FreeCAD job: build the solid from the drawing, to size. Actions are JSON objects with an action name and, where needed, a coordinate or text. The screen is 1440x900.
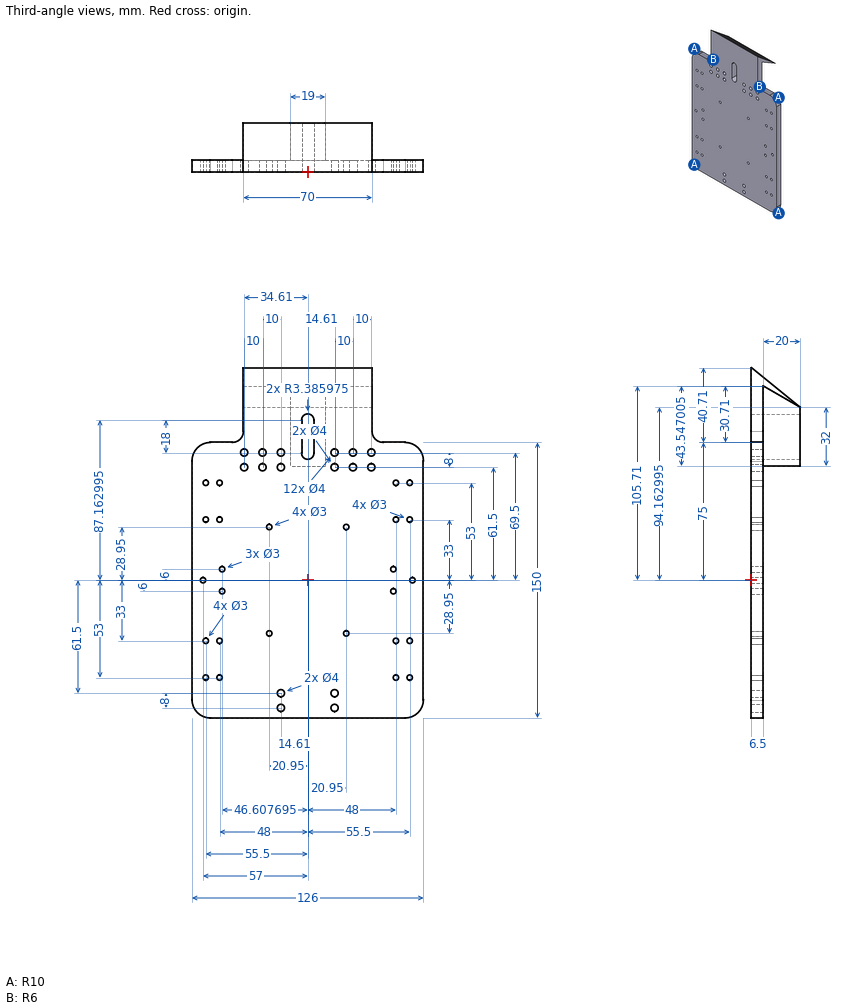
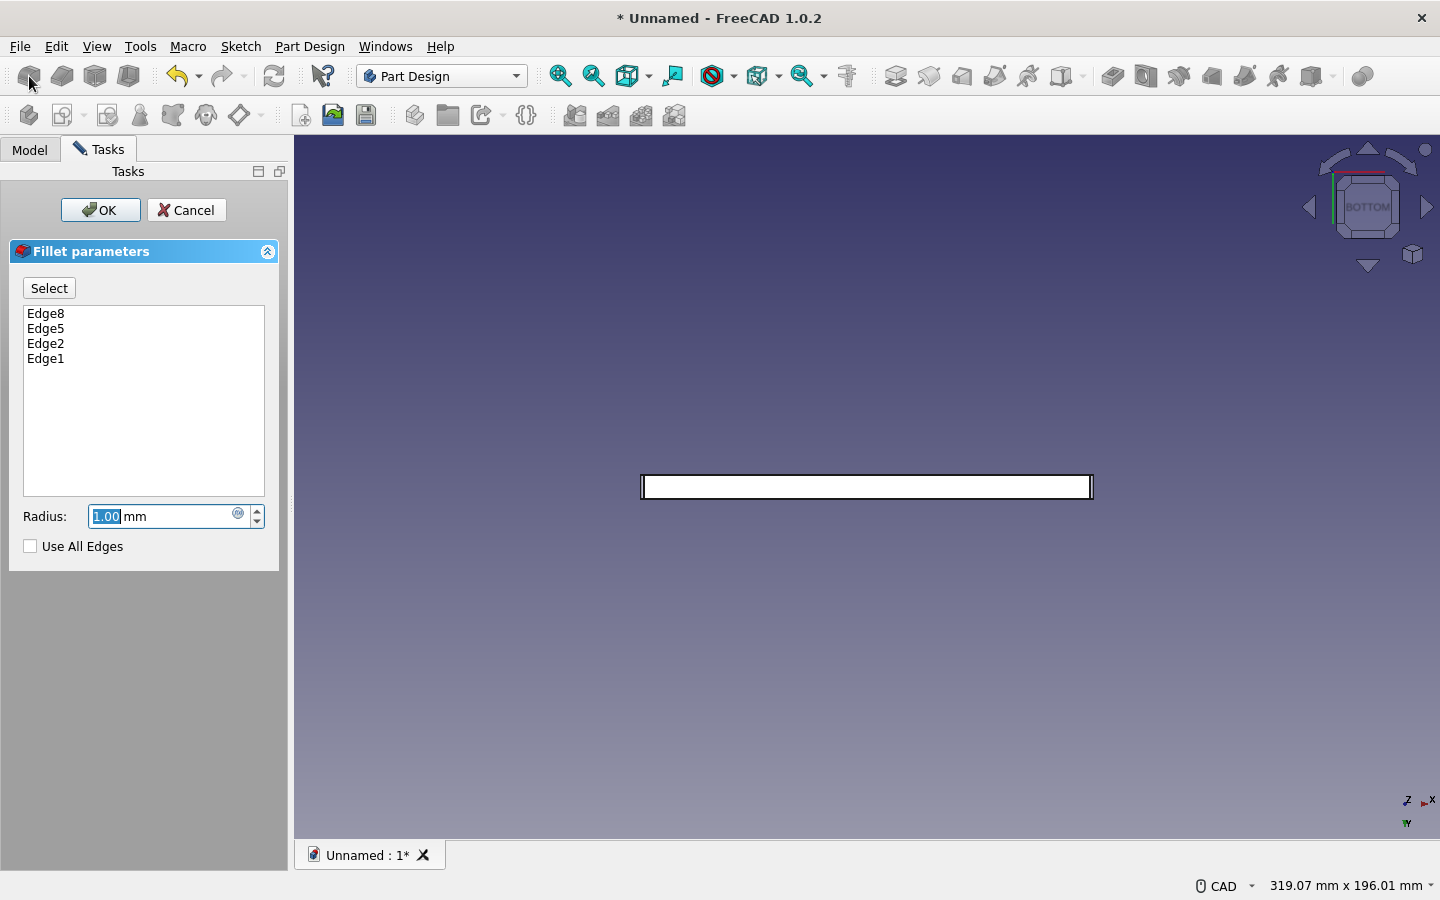
{"action": "type", "text": "10"}
{"action": "key", "text": "Tab"}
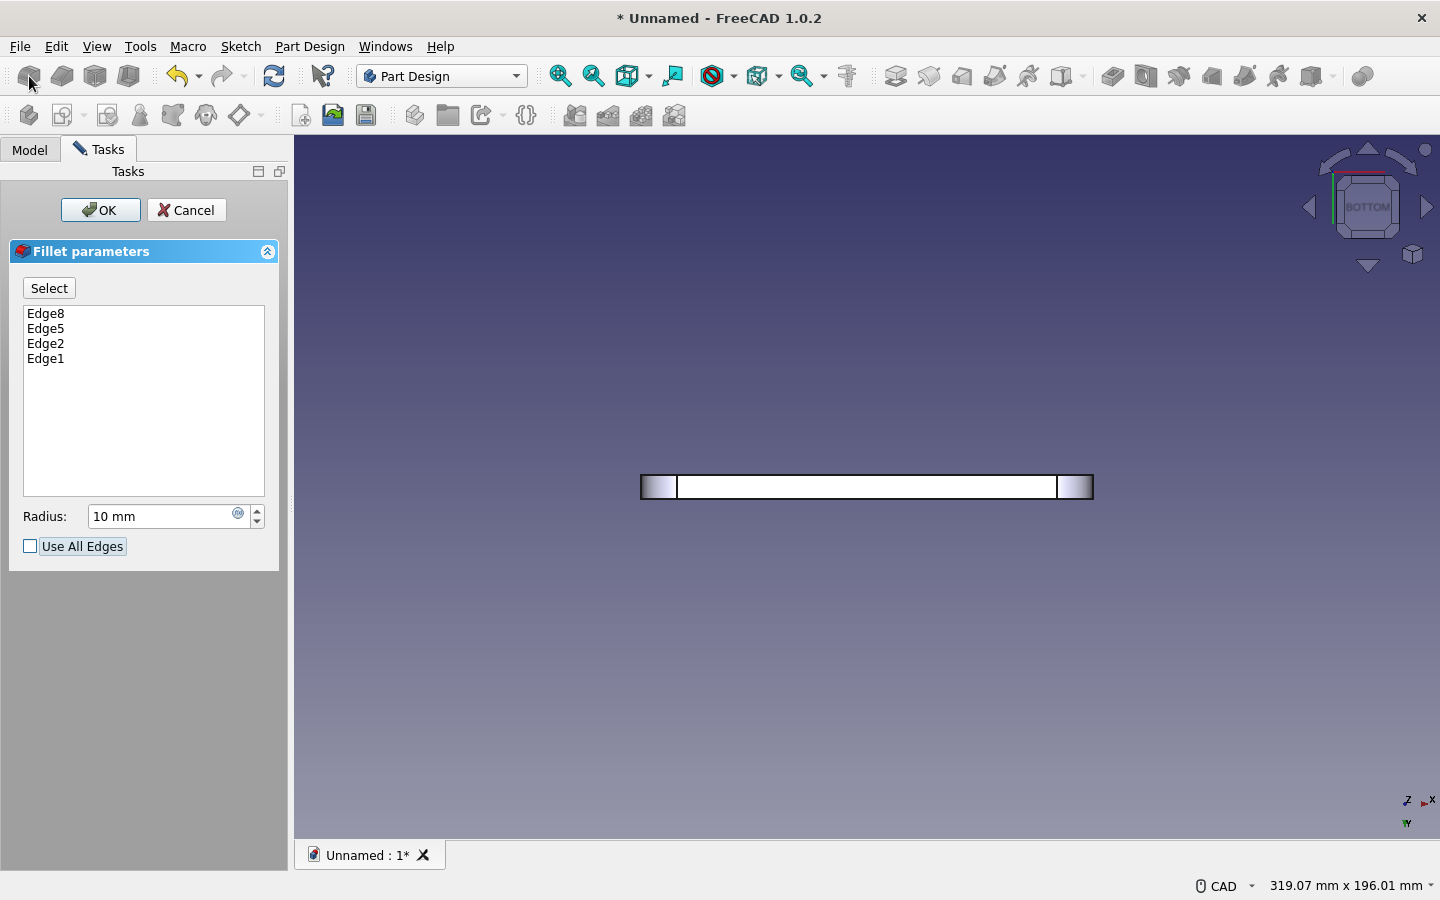
{"action": "left_click", "coordinate": [101, 210]}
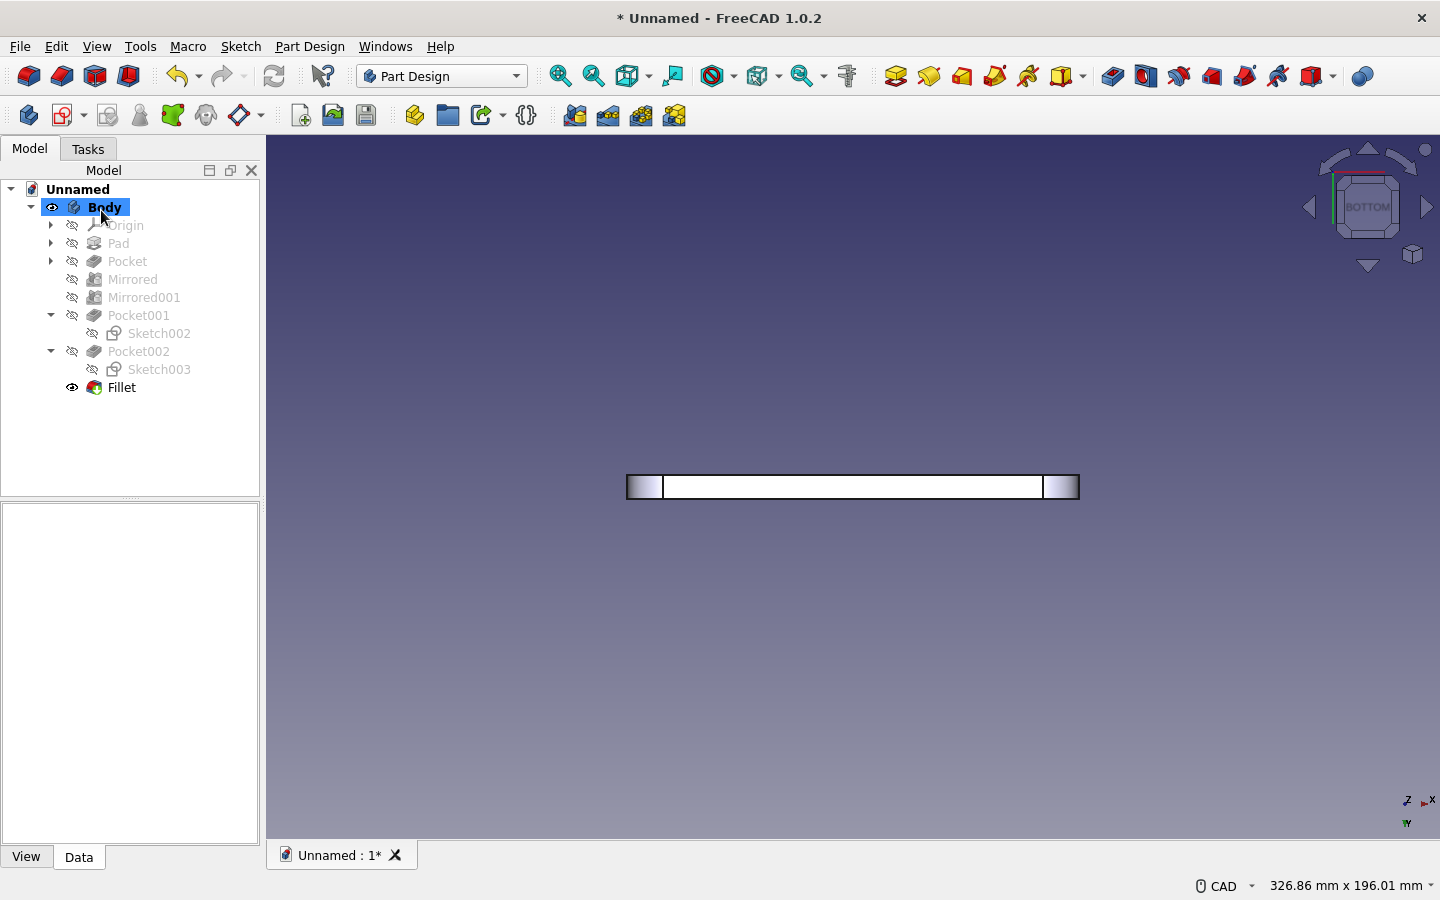
{"action": "left_click", "coordinate": [561, 76]}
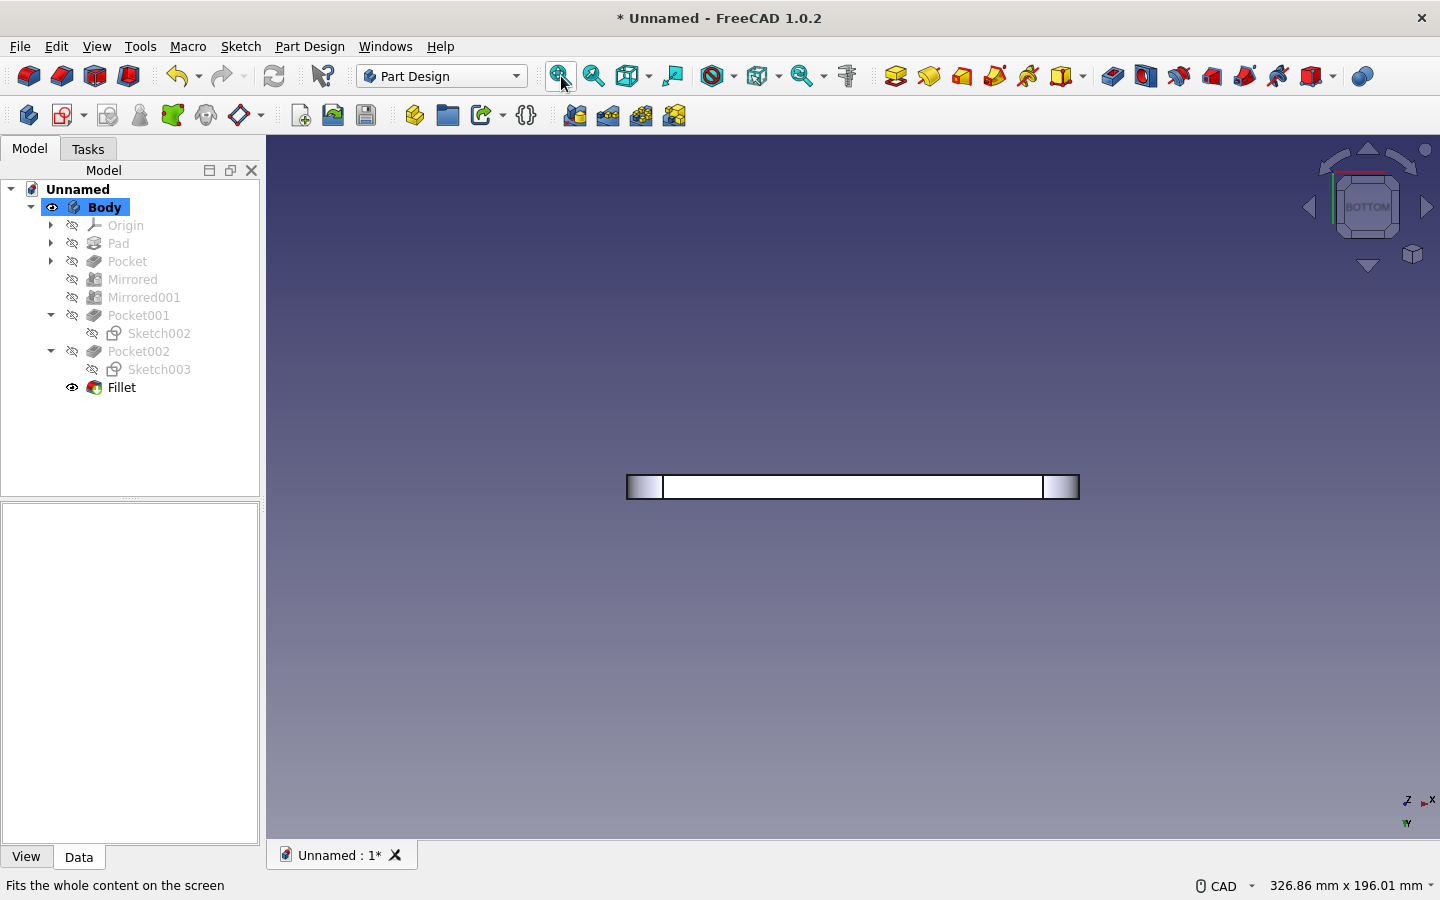
{"action": "key", "text": "4"}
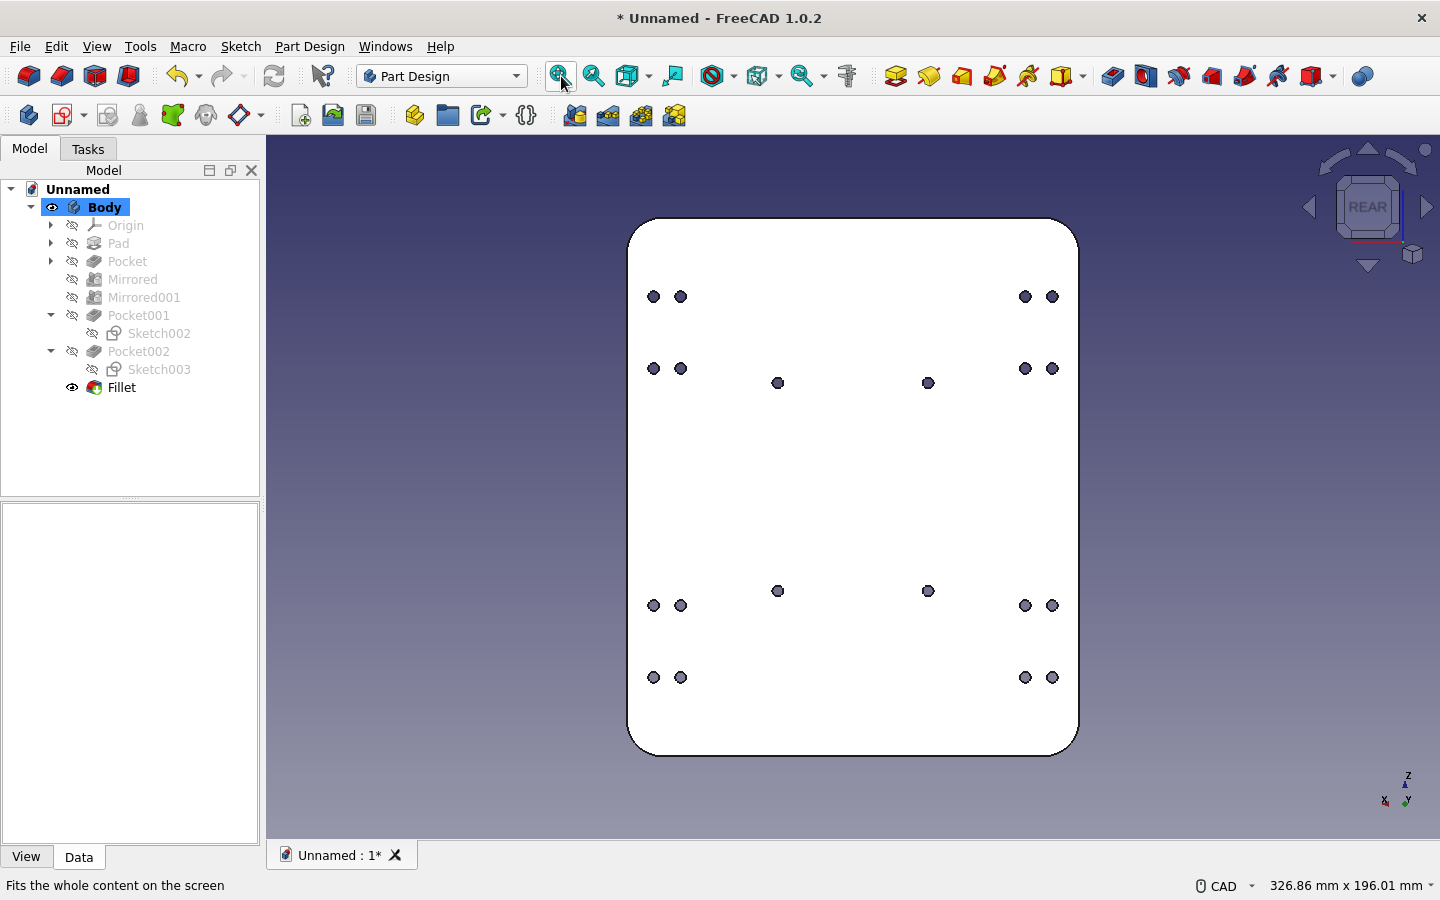
{"action": "left_click", "coordinate": [853, 486]}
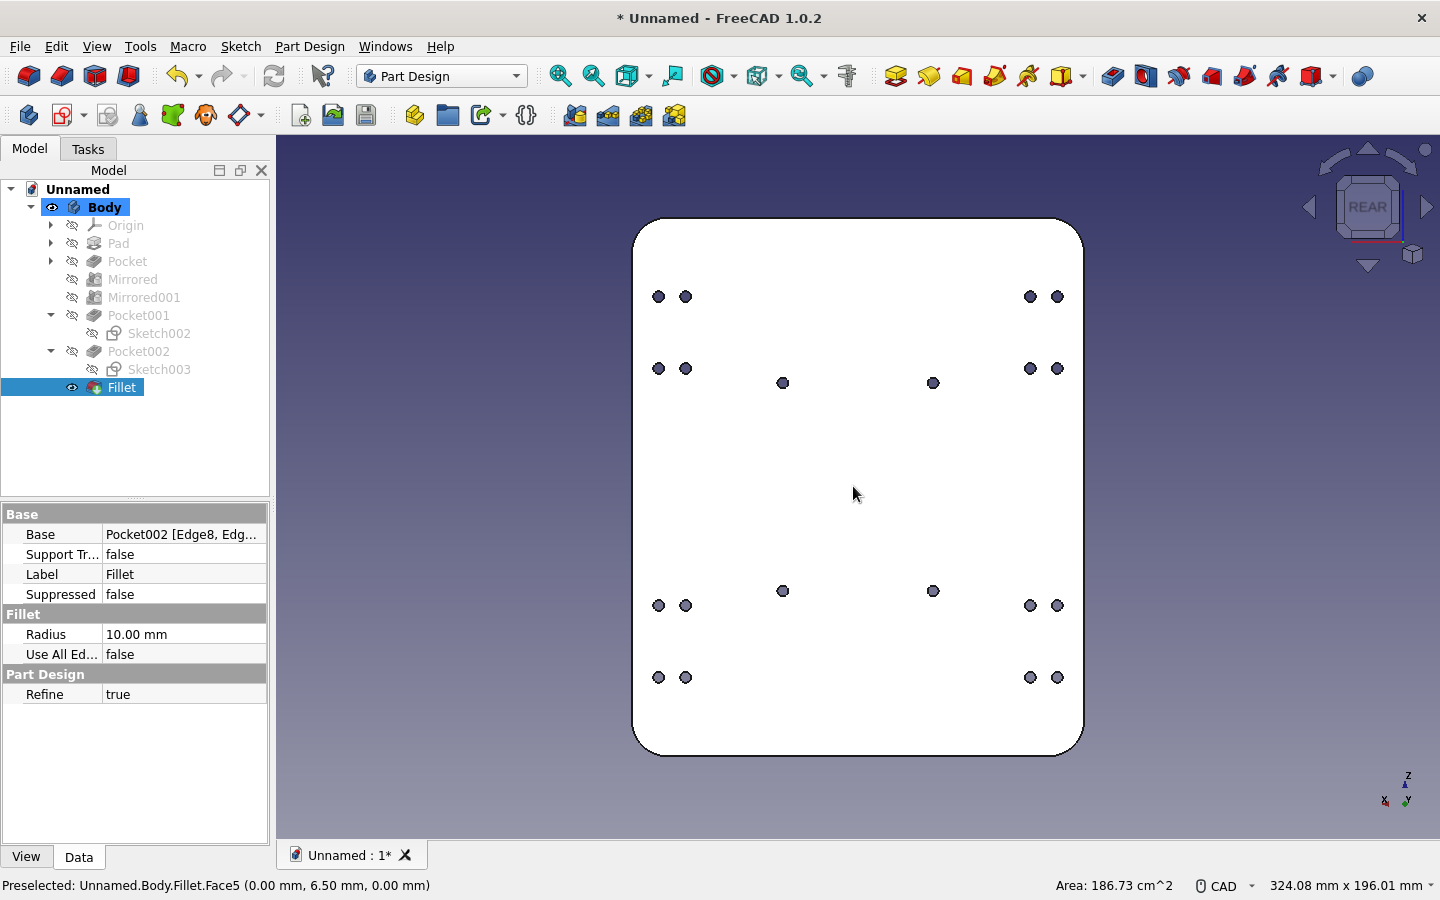
{"action": "left_click", "coordinate": [62, 116]}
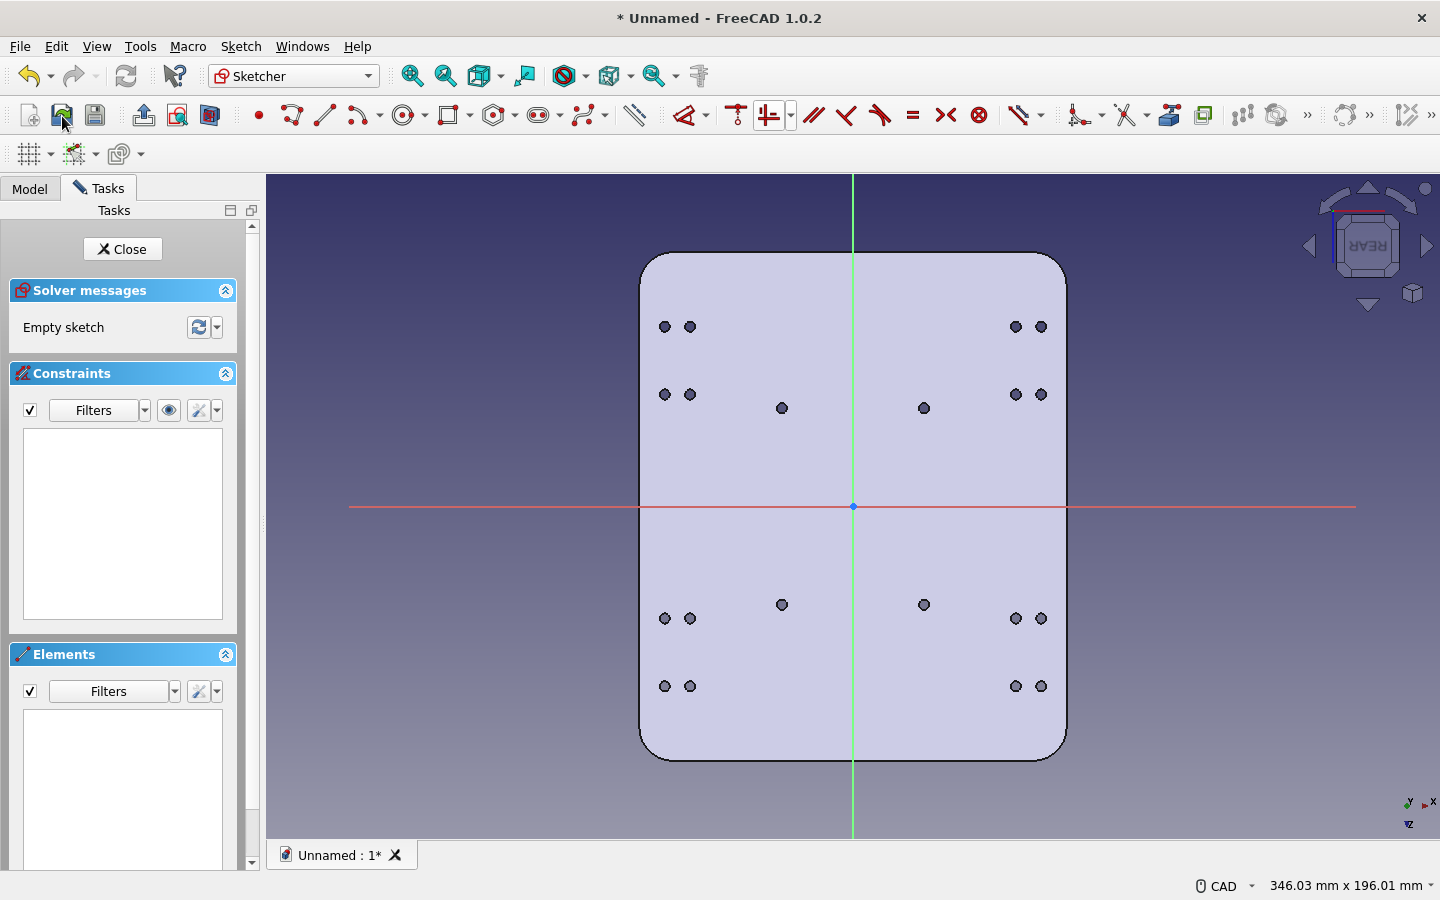
{"action": "scroll", "coordinate": [664, 507], "scroll_direction": "up", "scroll_amount": 11}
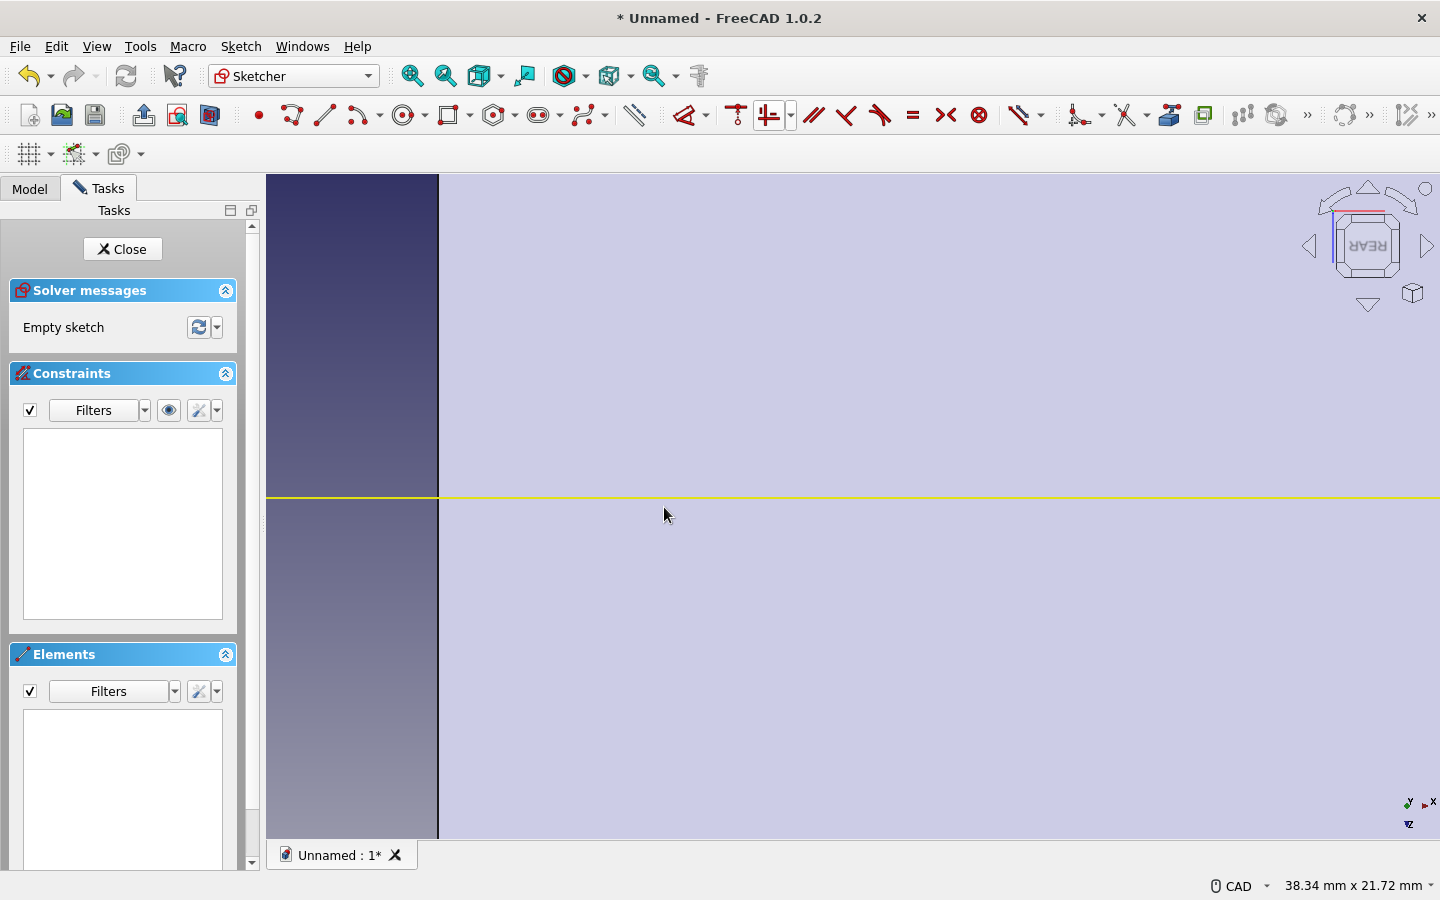
{"action": "left_click", "coordinate": [402, 116]}